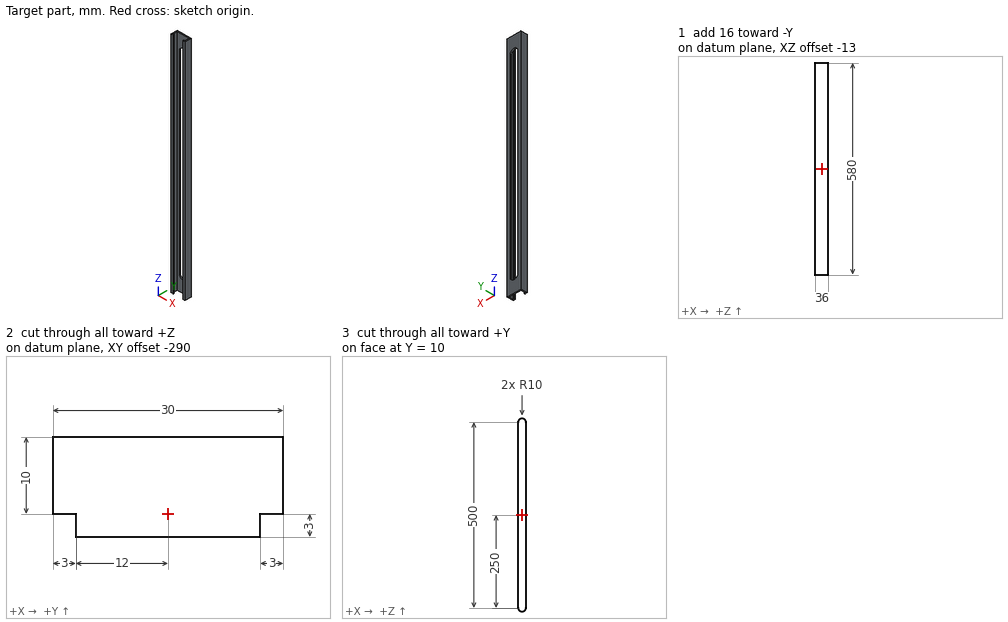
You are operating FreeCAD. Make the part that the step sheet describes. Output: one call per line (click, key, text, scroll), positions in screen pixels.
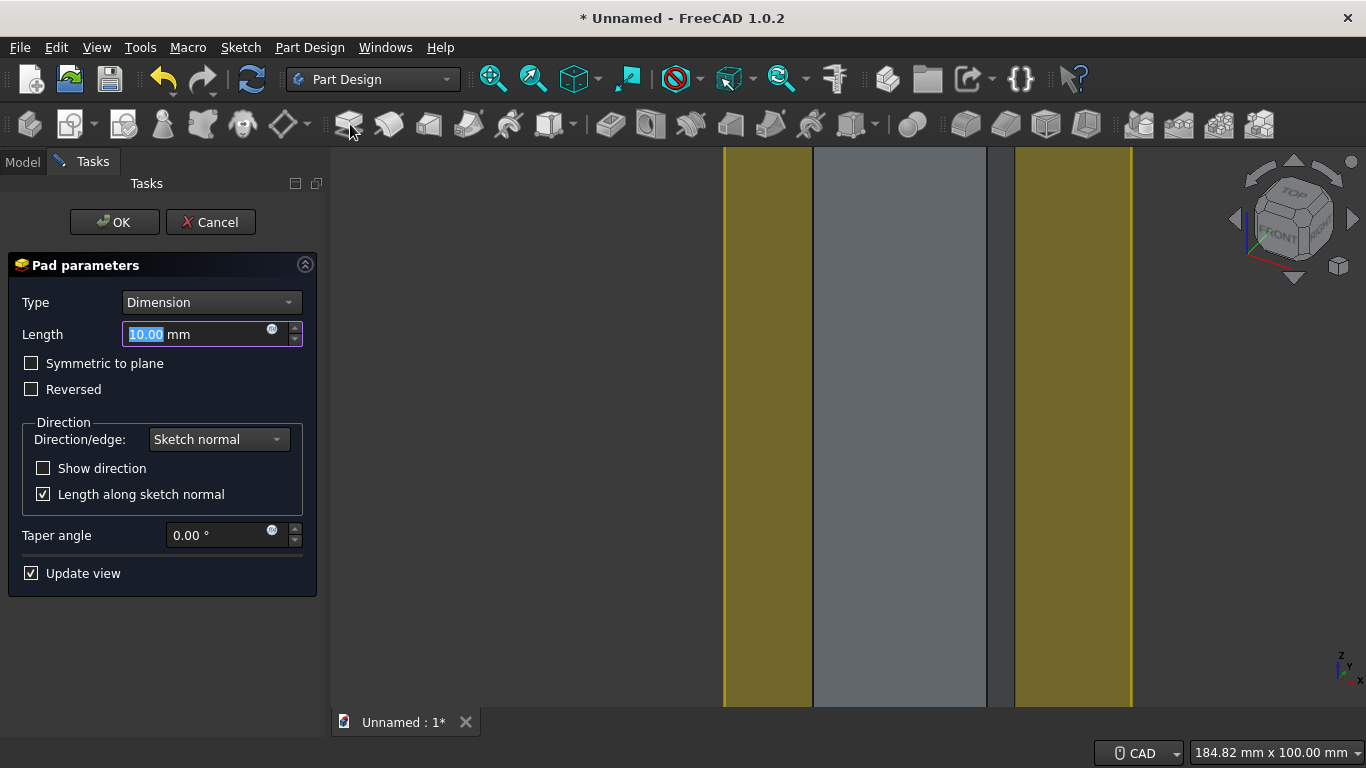
text(16)
key(Tab)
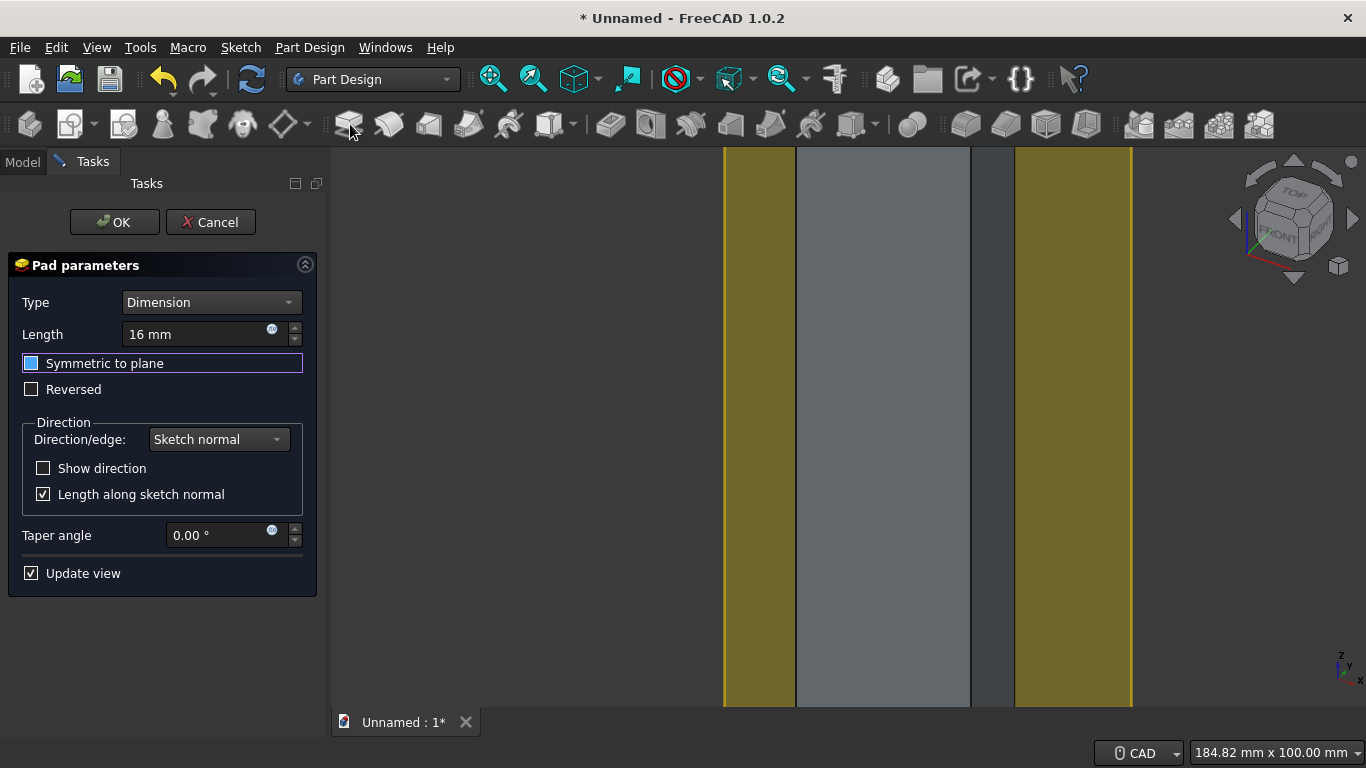
click(115, 222)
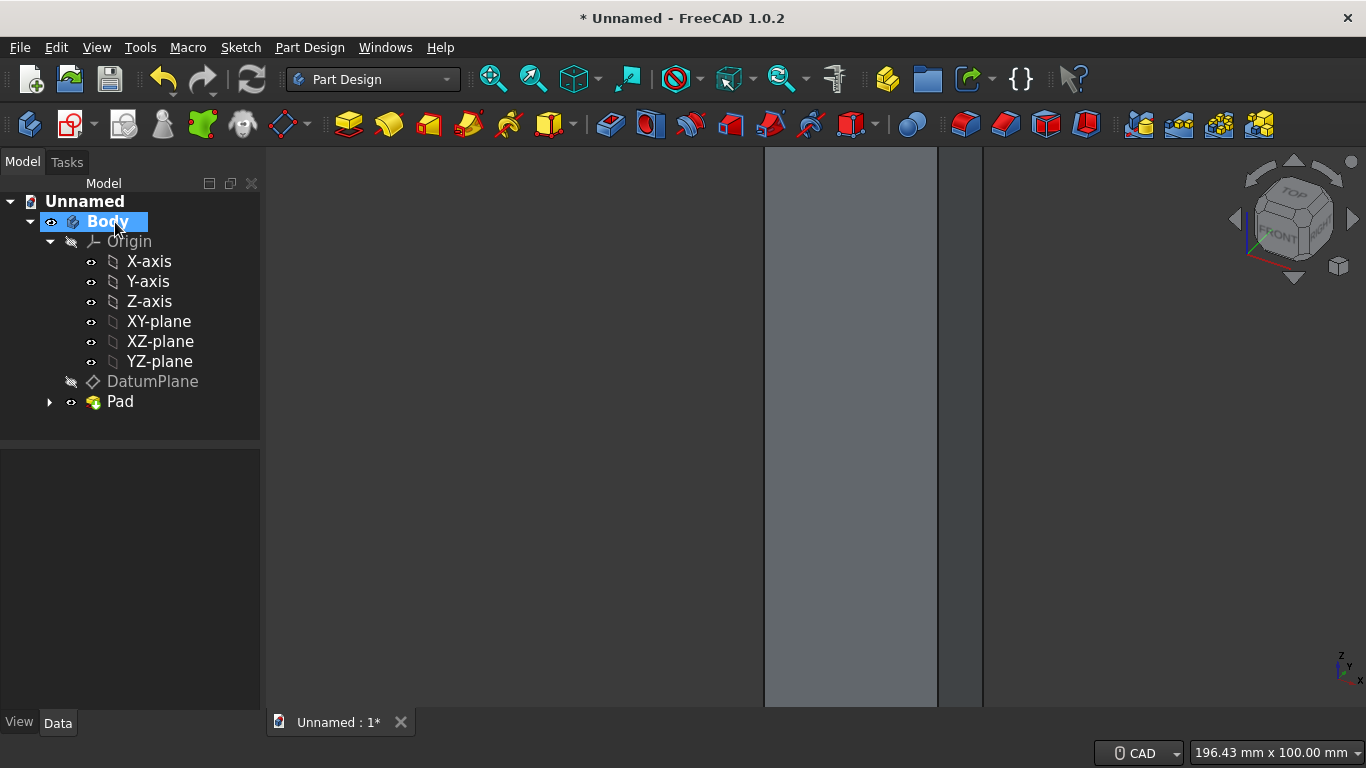
click(494, 80)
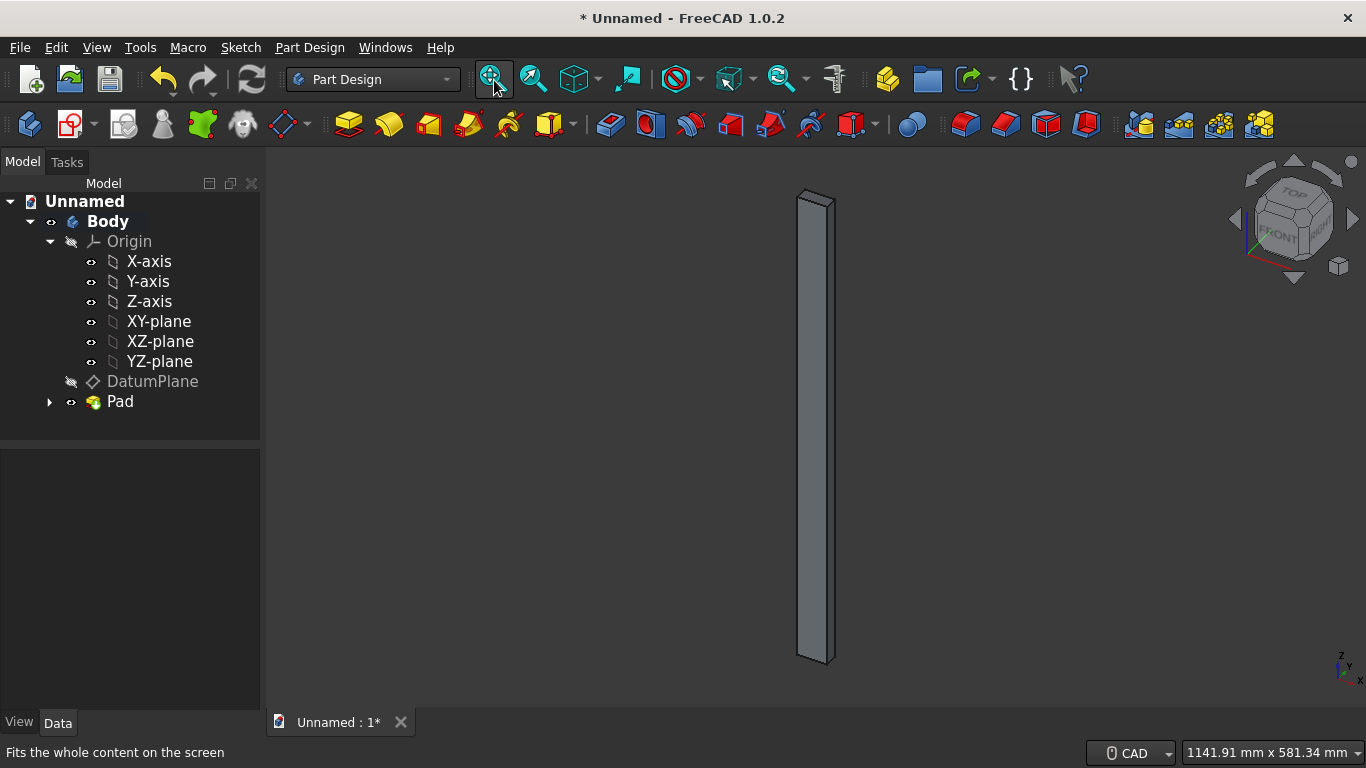
key(5)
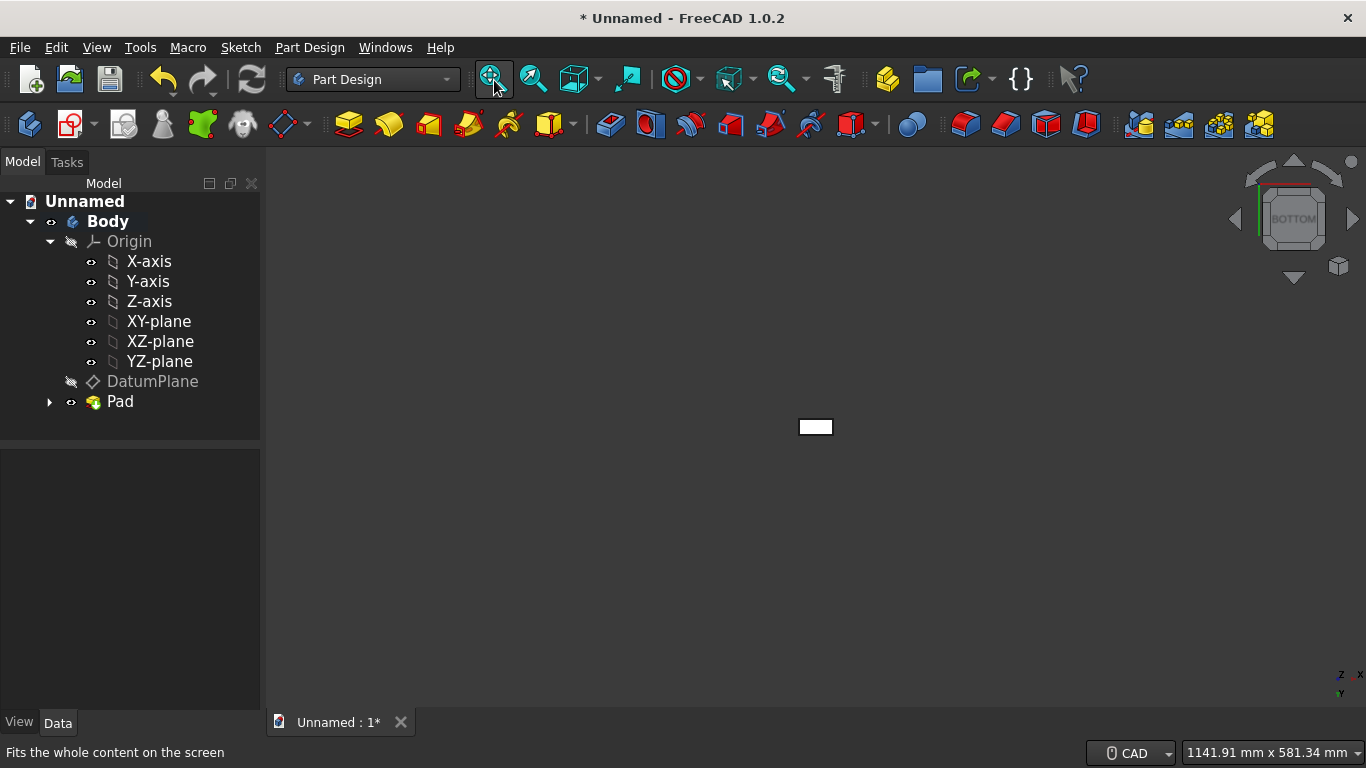
click(494, 80)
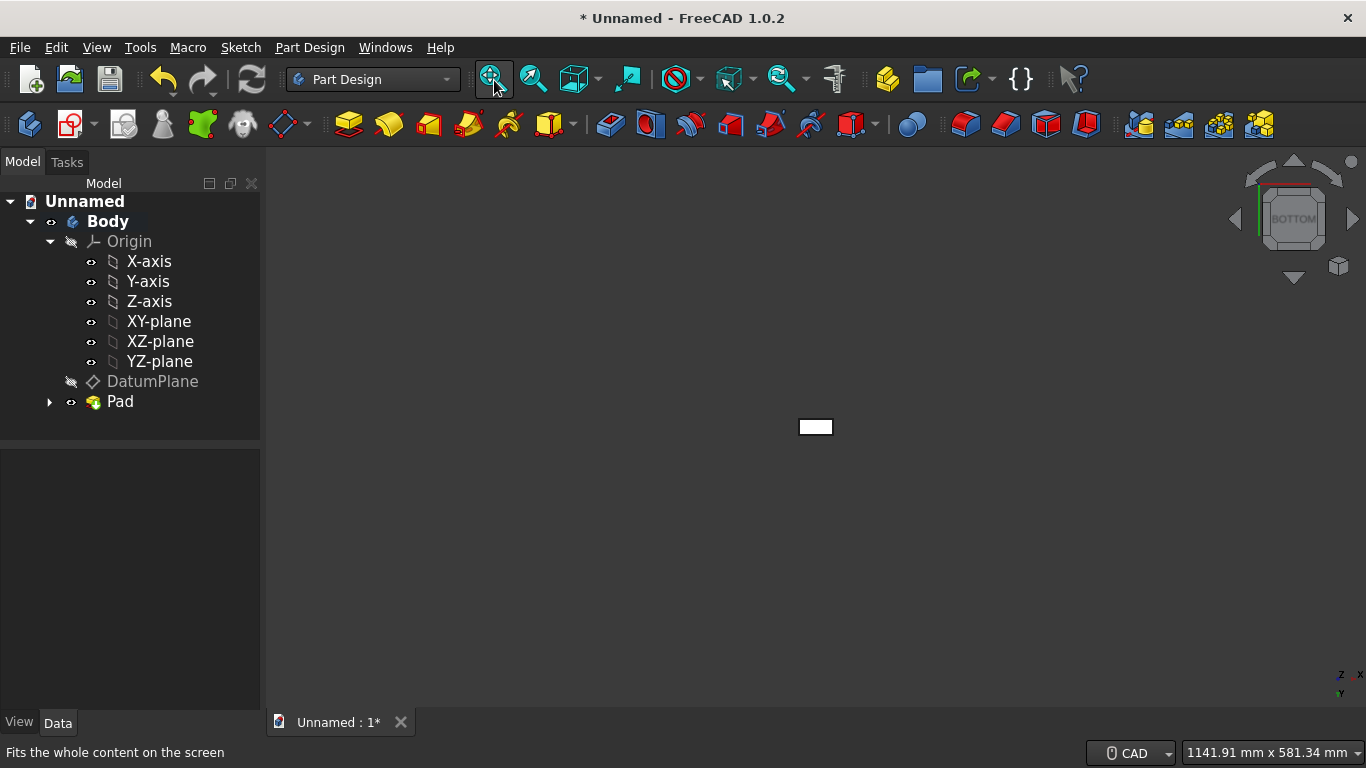
key(1)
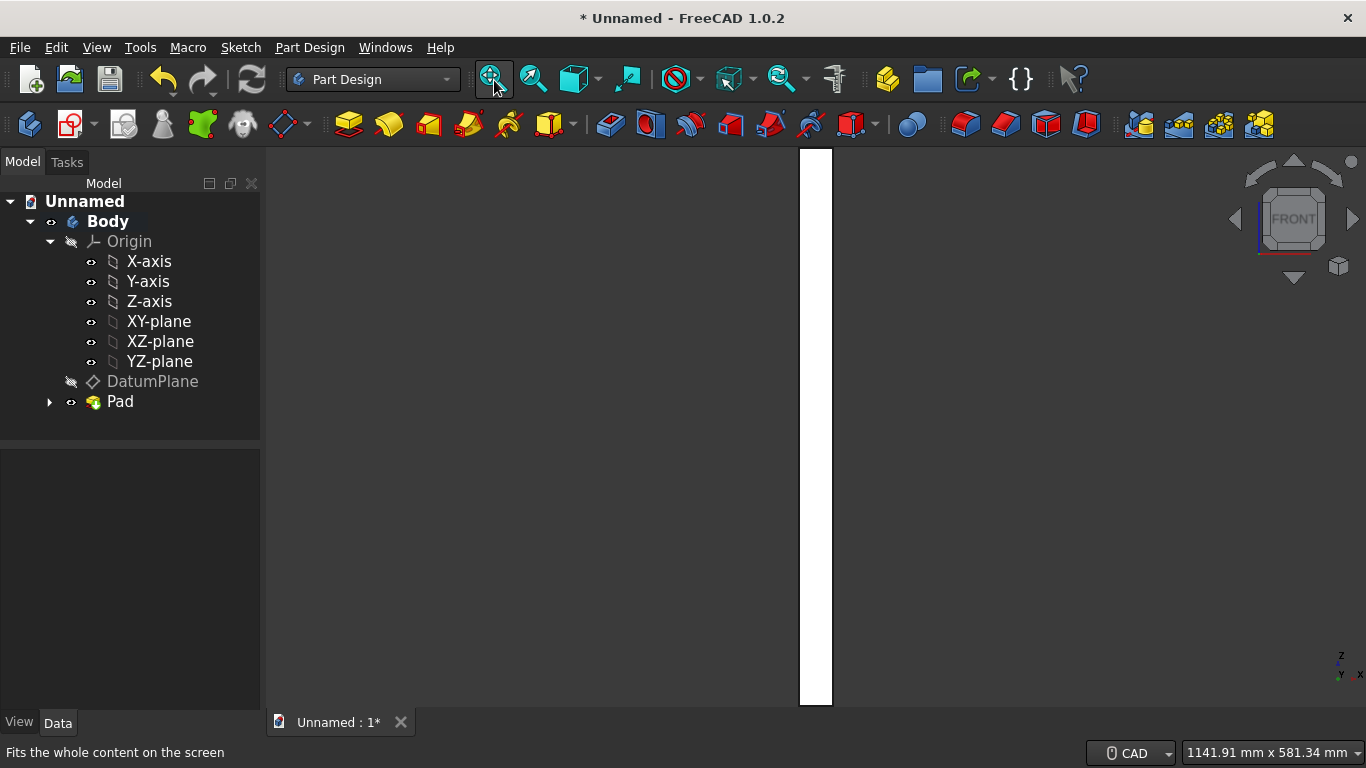
key(3)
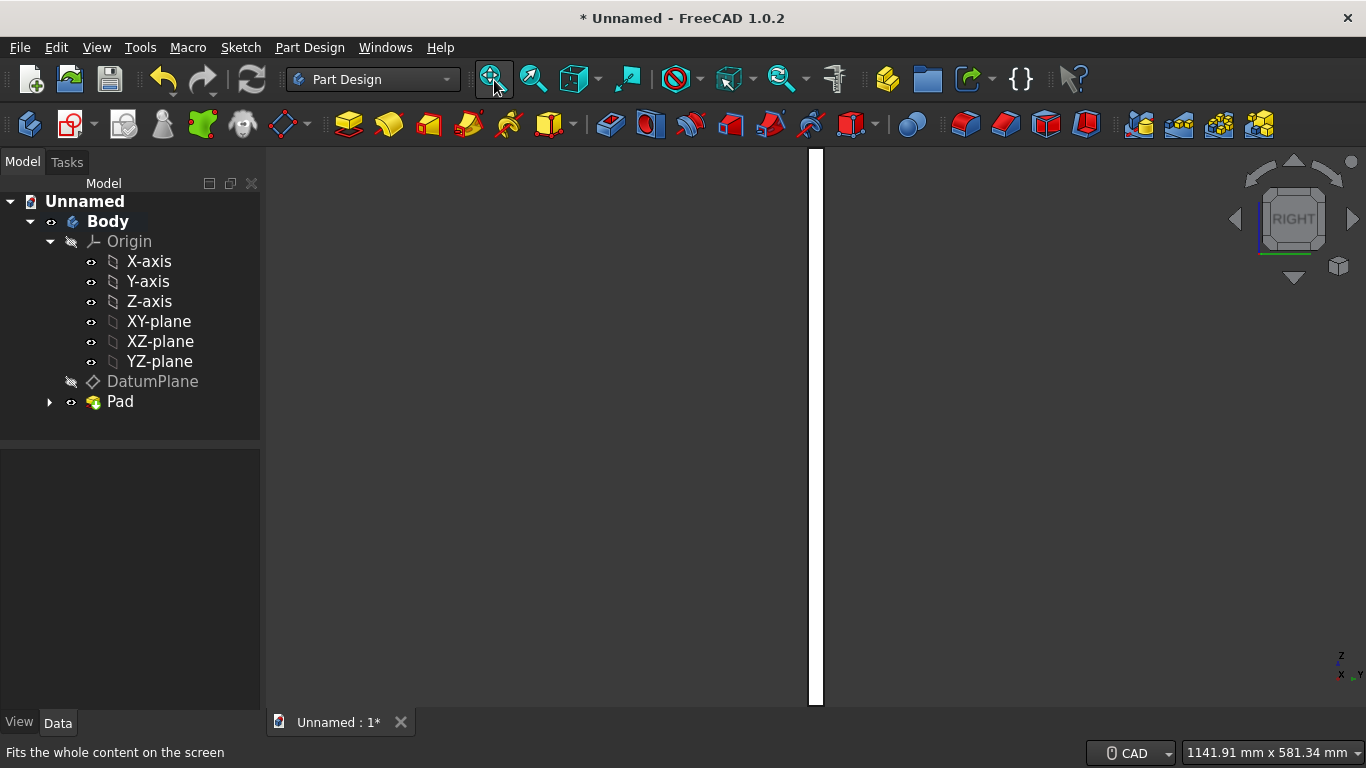
click(136, 322)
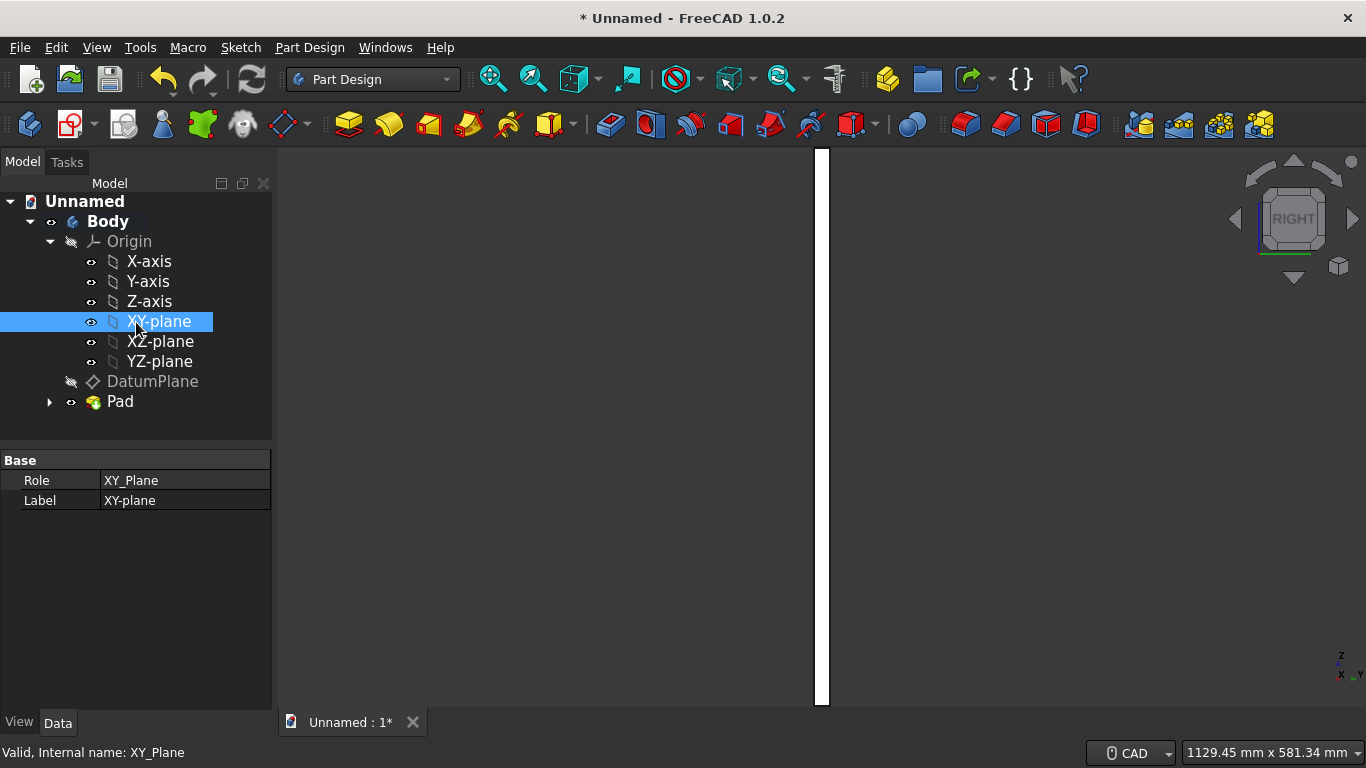
click(284, 124)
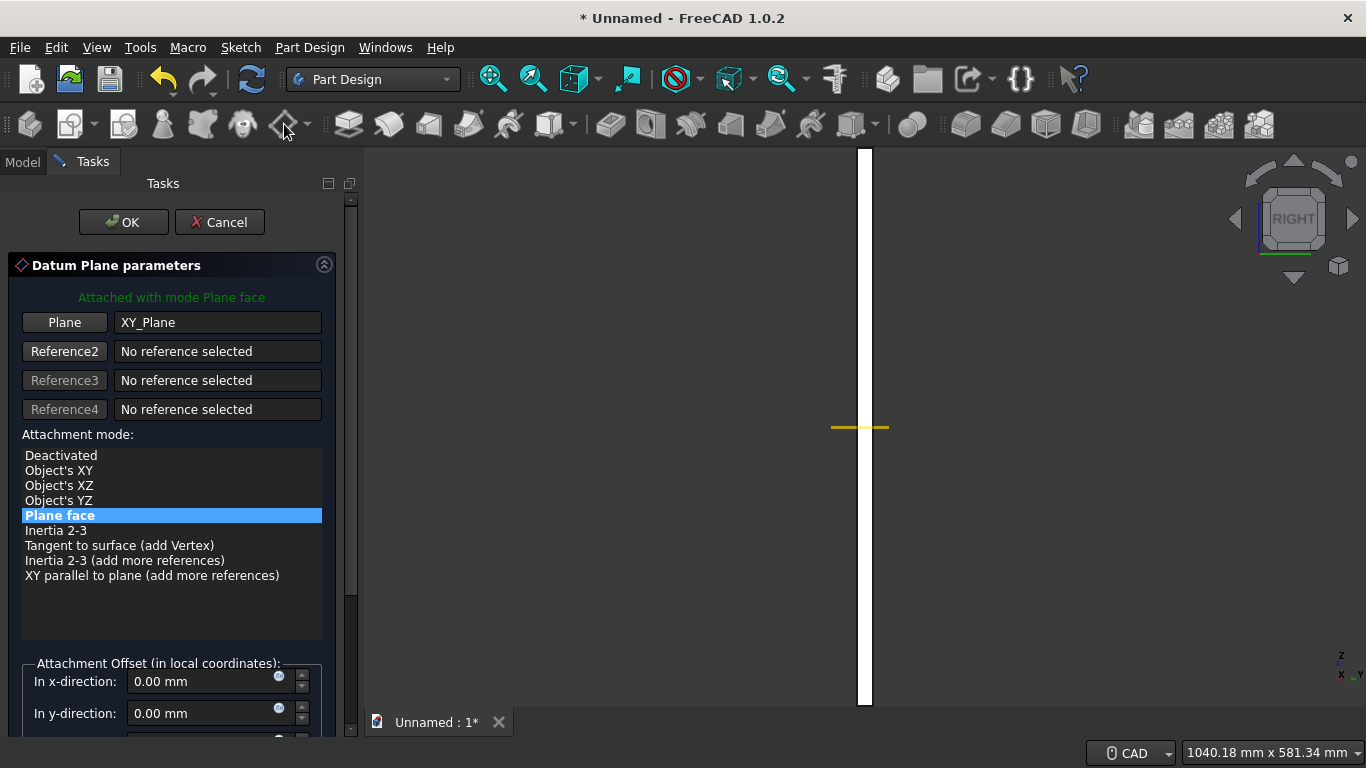
scroll(351, 464, down, 2)